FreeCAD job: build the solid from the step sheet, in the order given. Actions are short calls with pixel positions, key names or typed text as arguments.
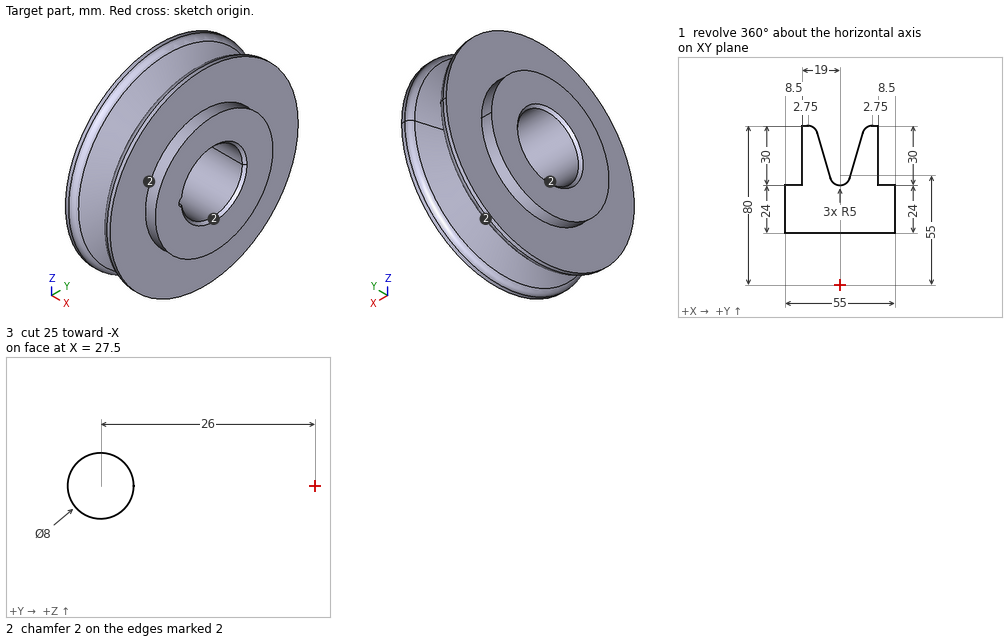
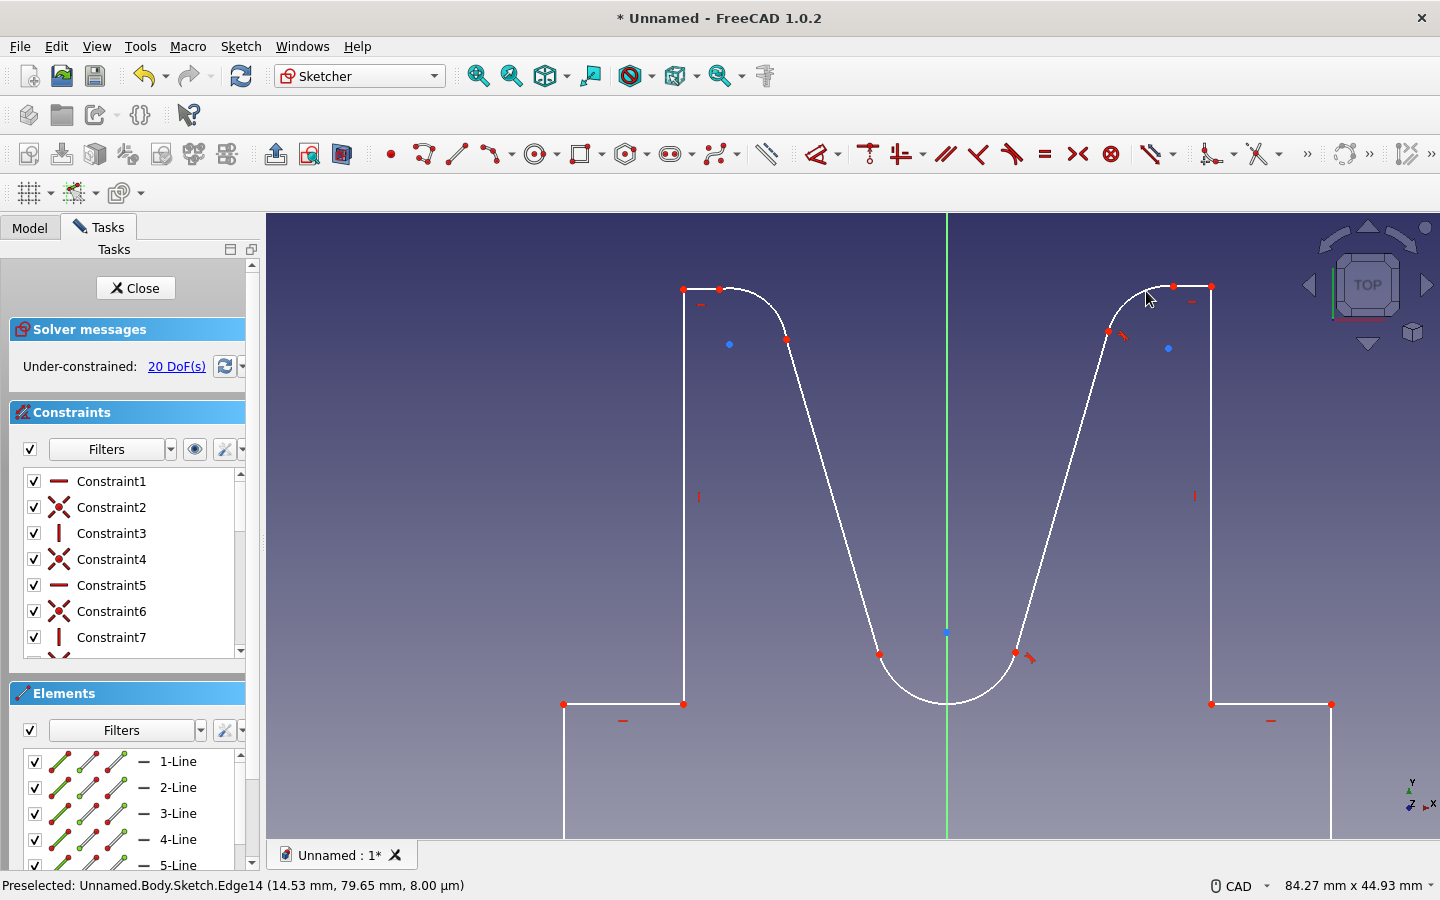
click(851, 560)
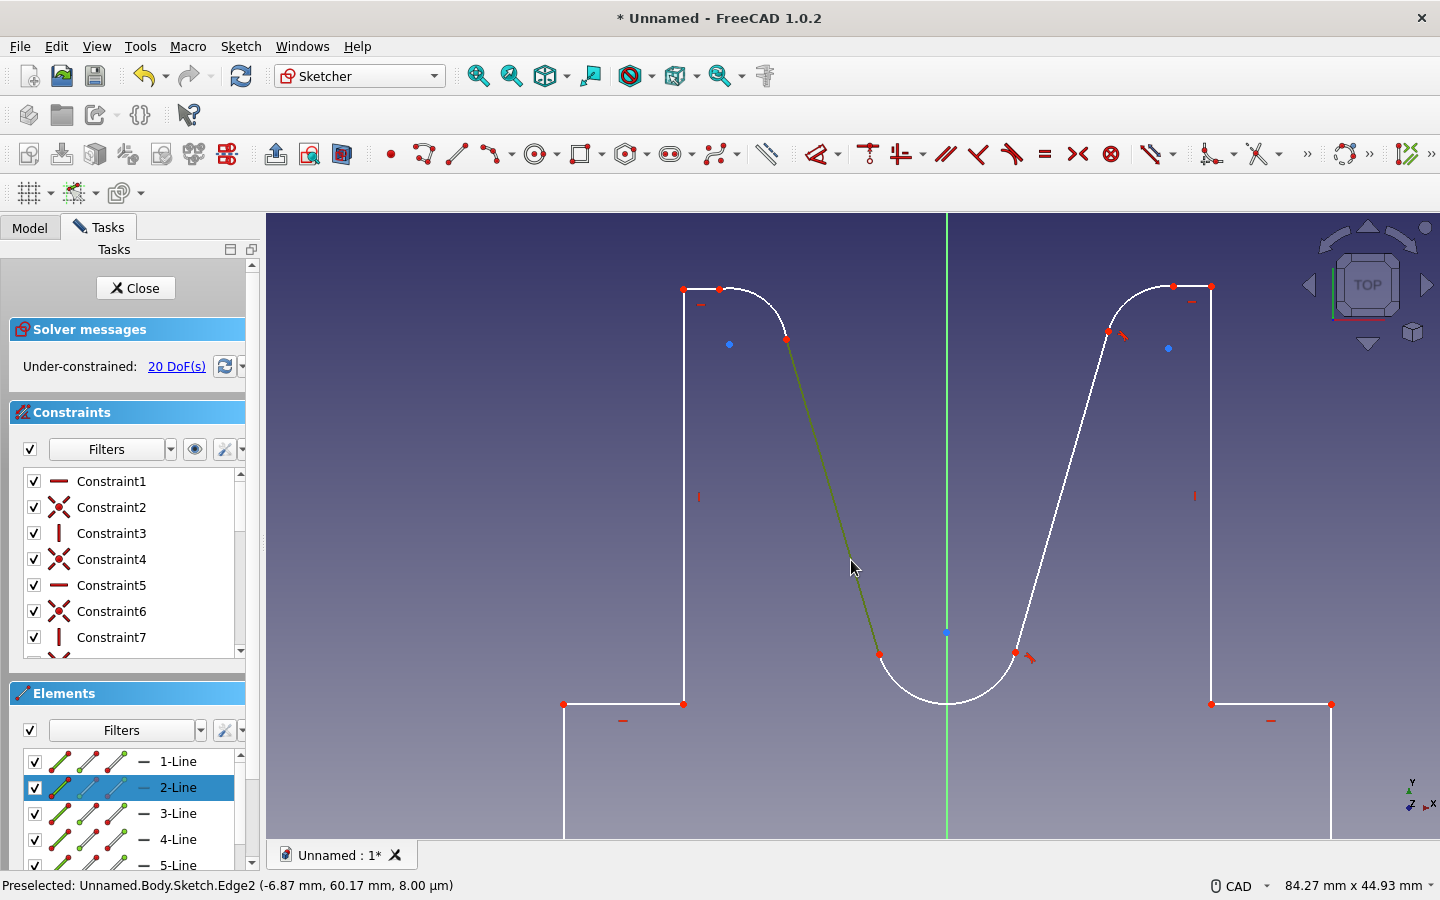
click(913, 695)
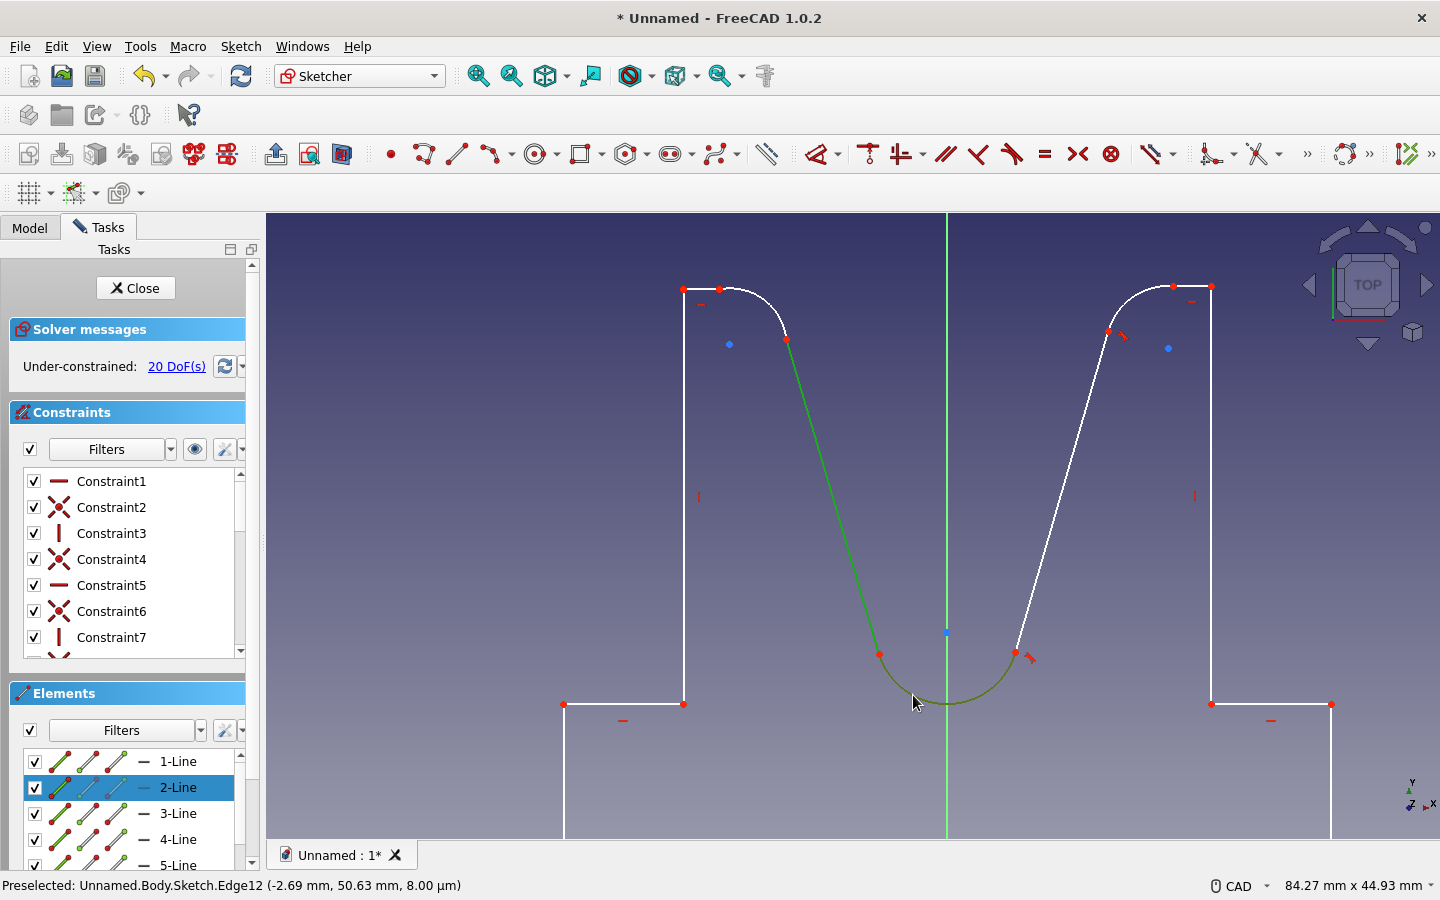
click(1012, 154)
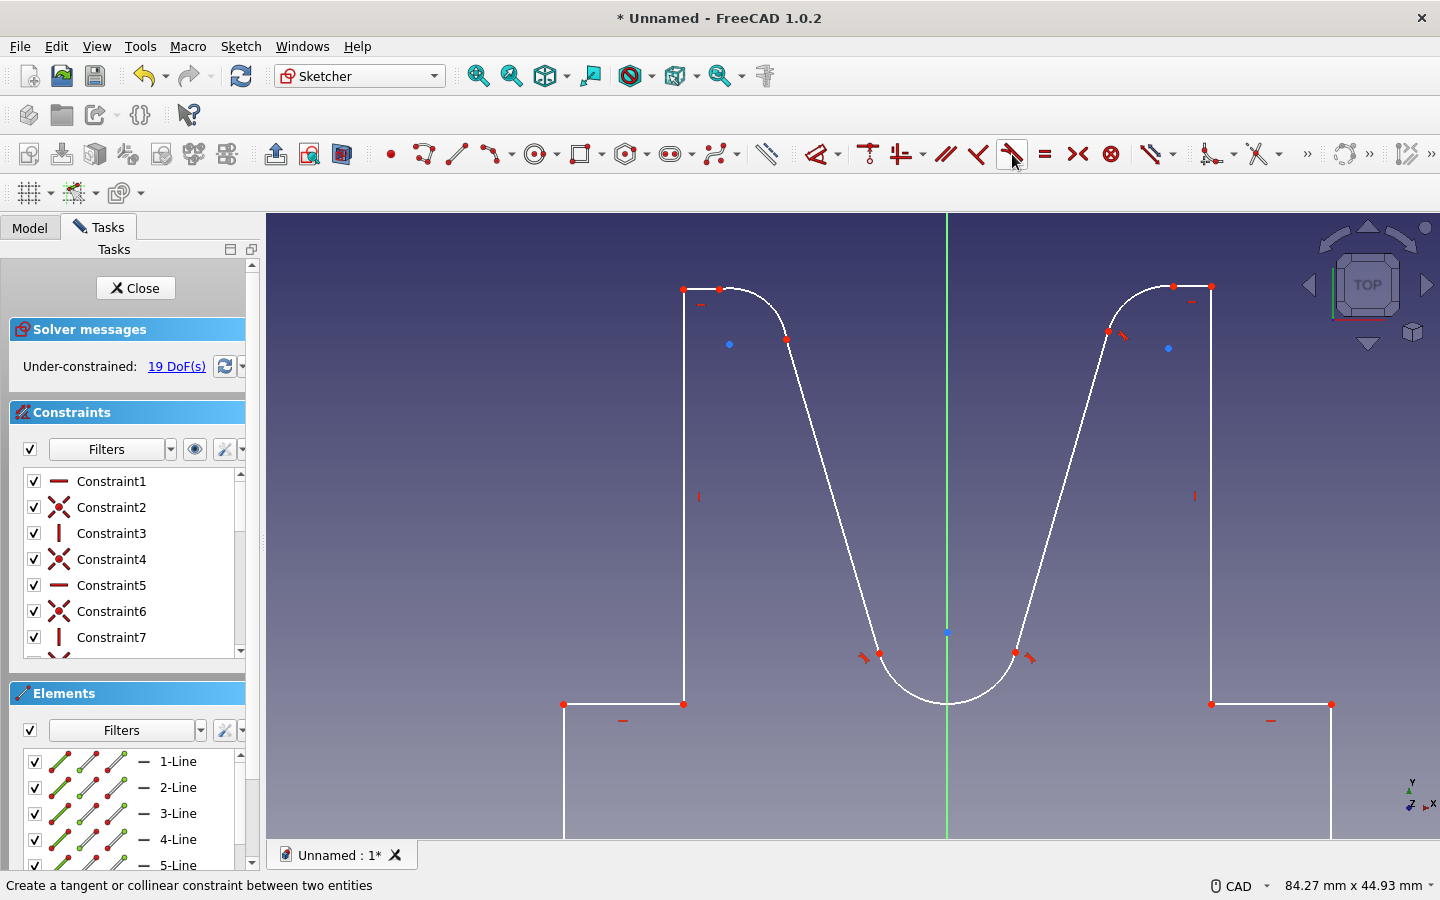
click(851, 559)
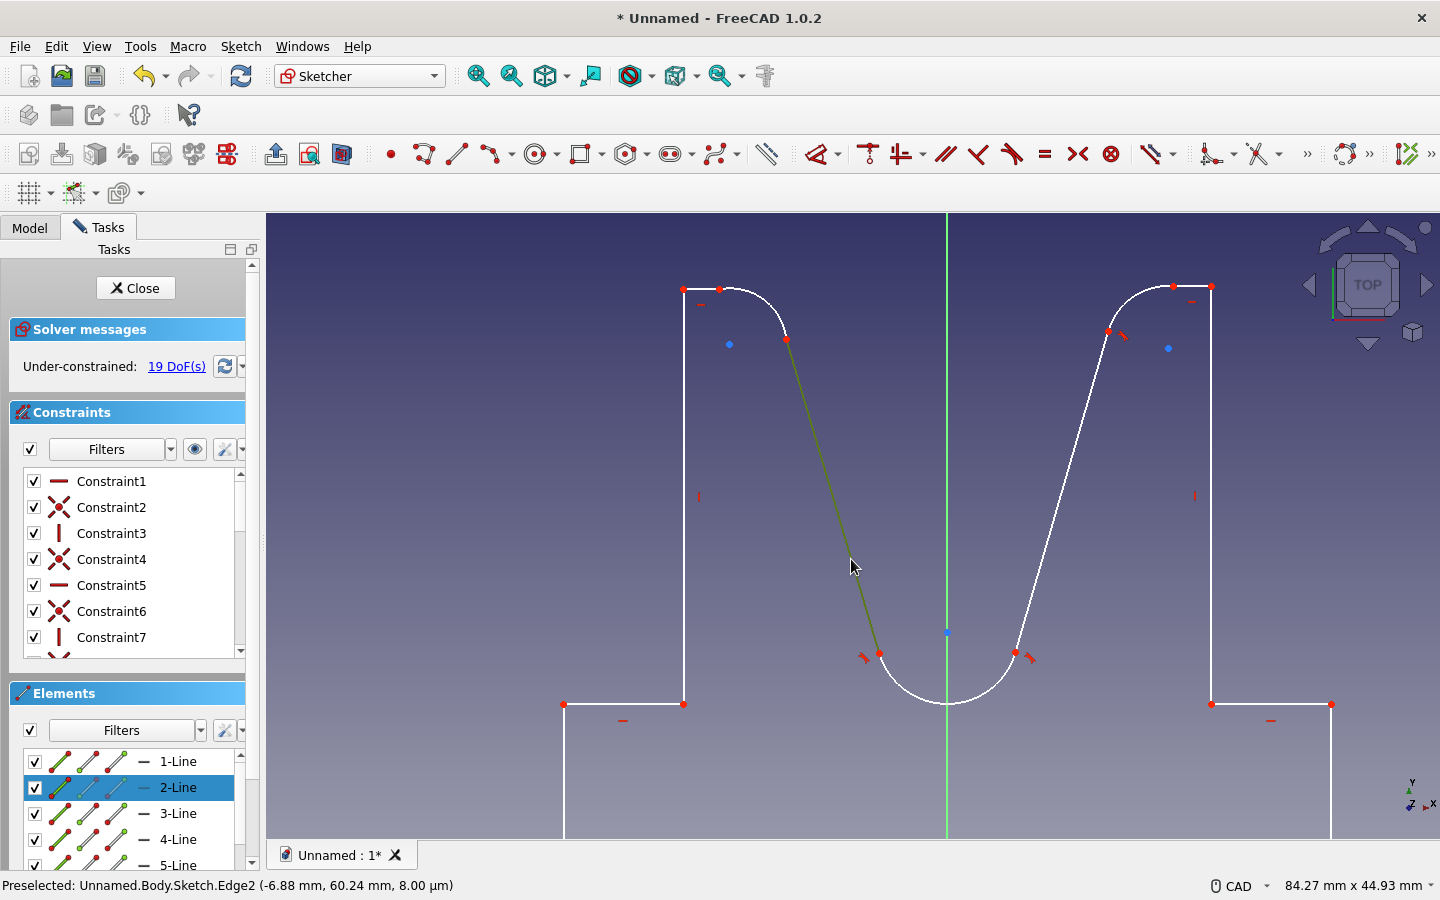
click(777, 313)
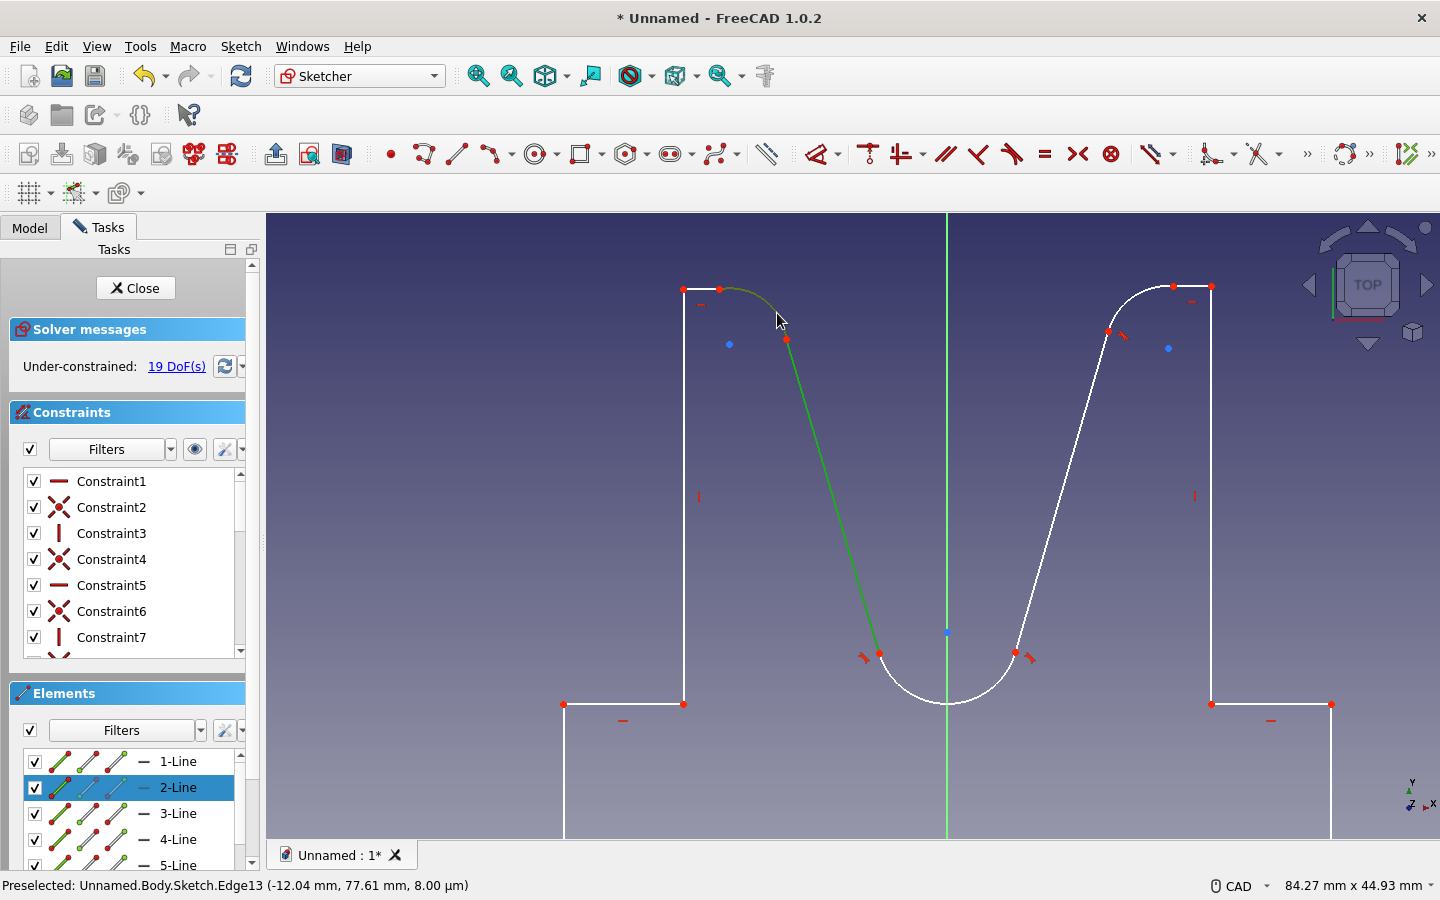
key(t)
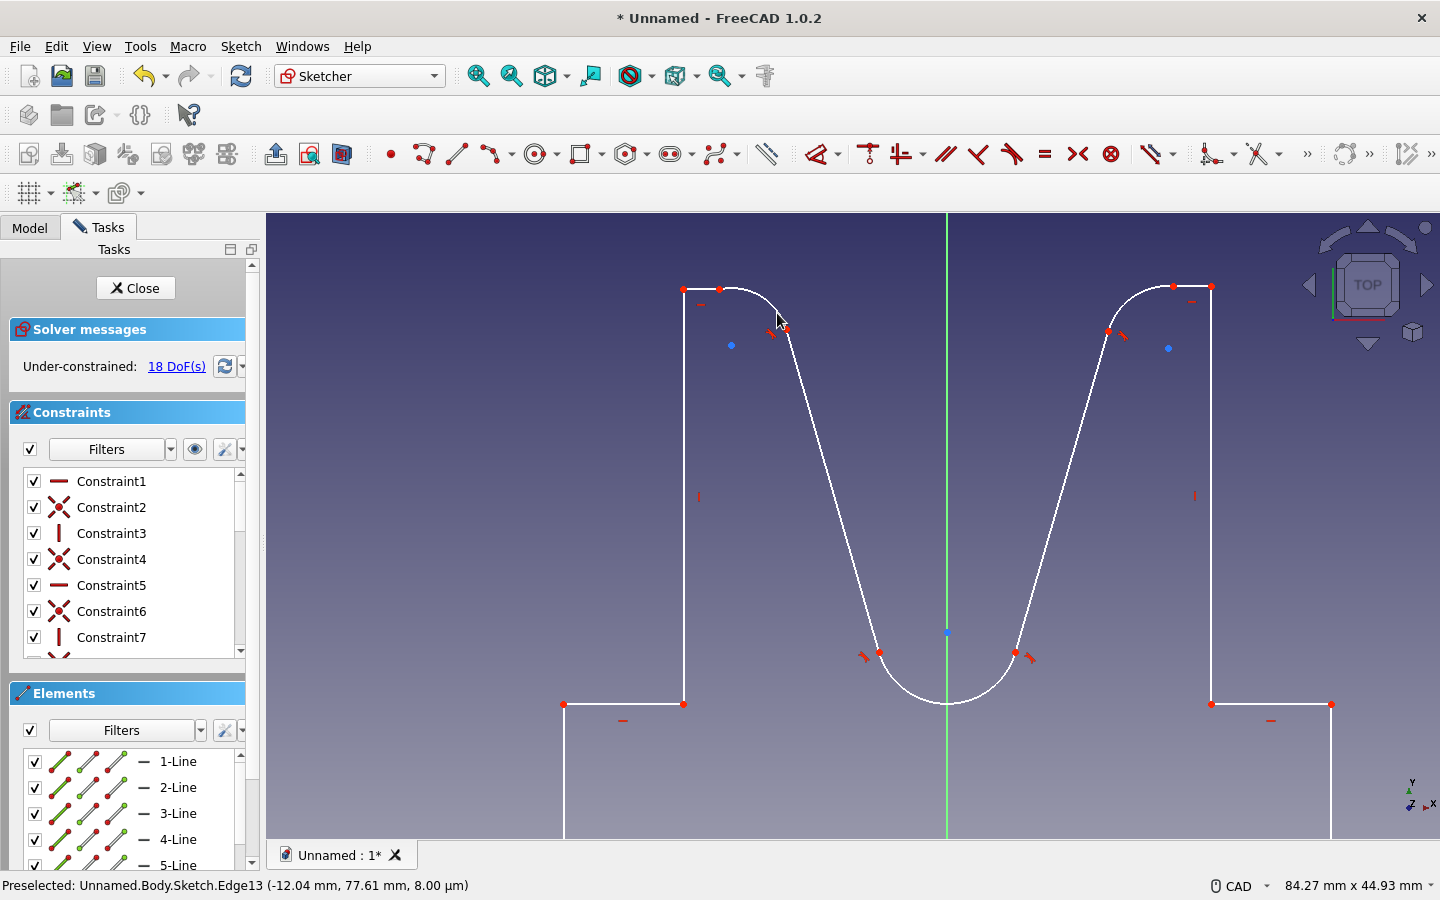
scroll(709, 289, up, 2)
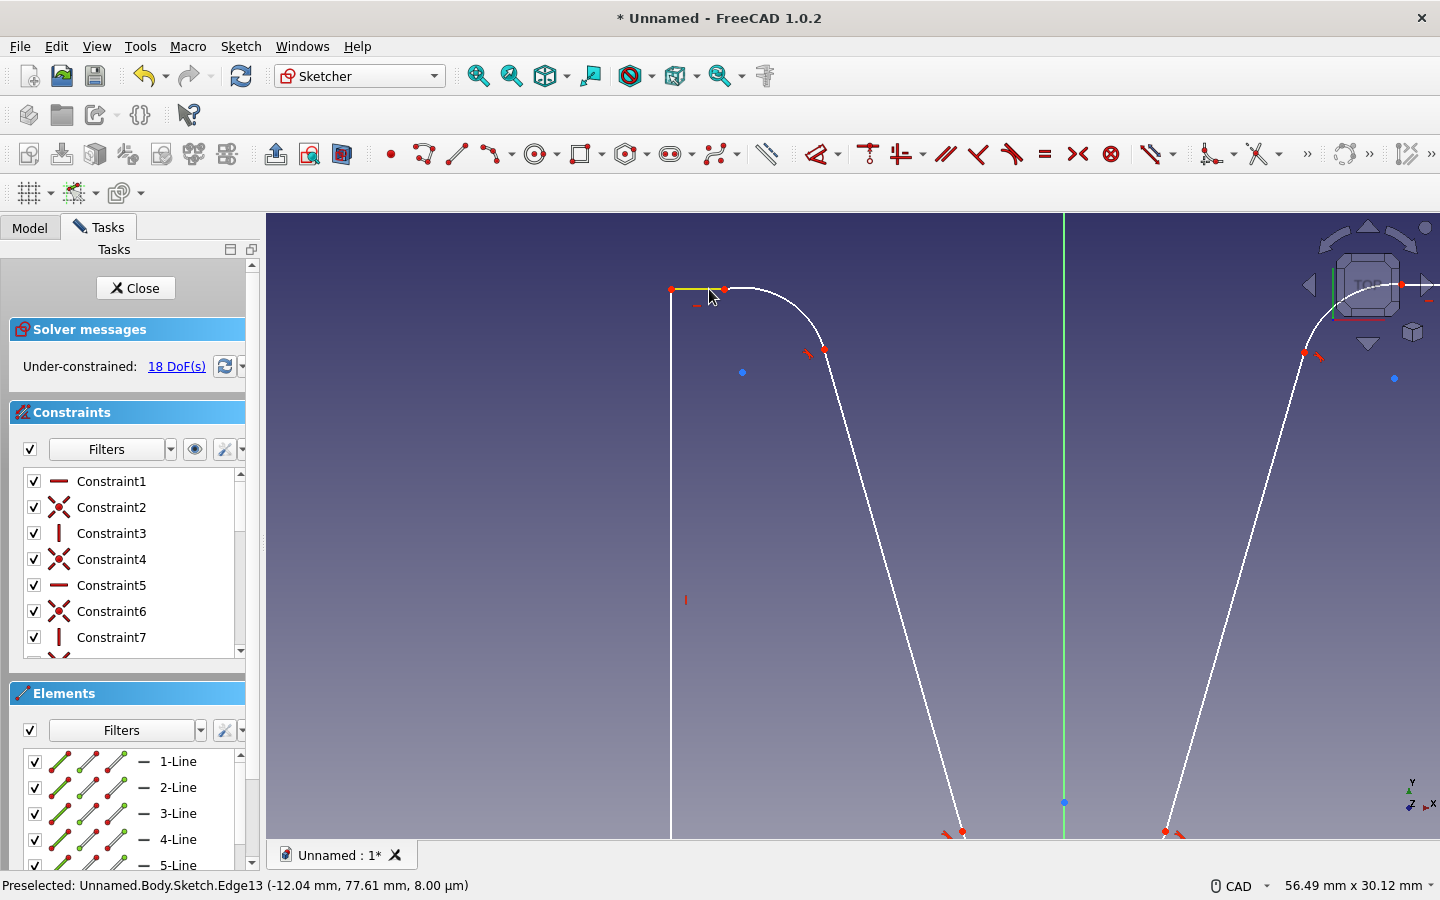
click(709, 289)